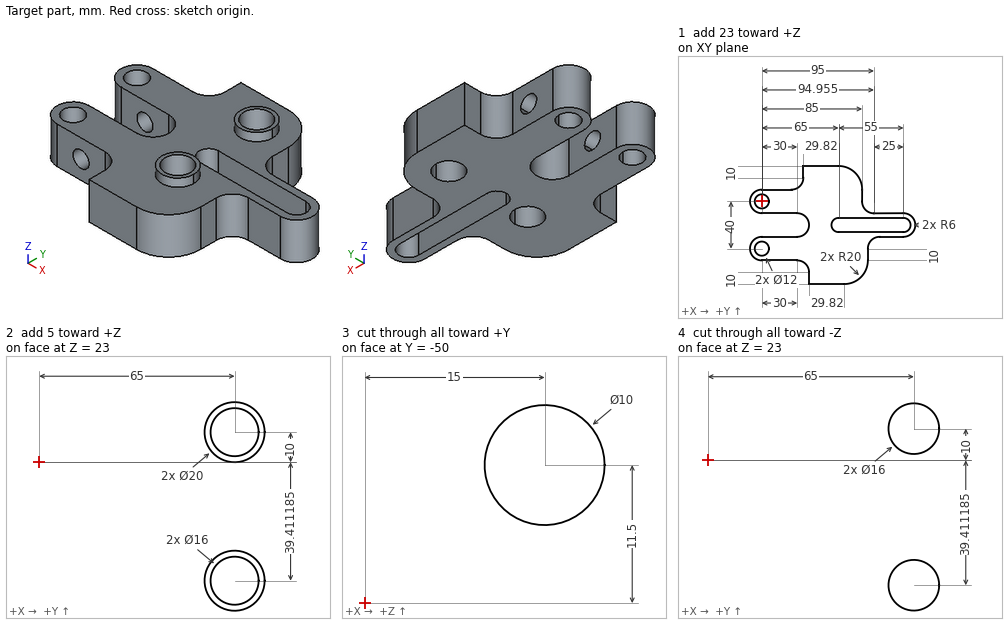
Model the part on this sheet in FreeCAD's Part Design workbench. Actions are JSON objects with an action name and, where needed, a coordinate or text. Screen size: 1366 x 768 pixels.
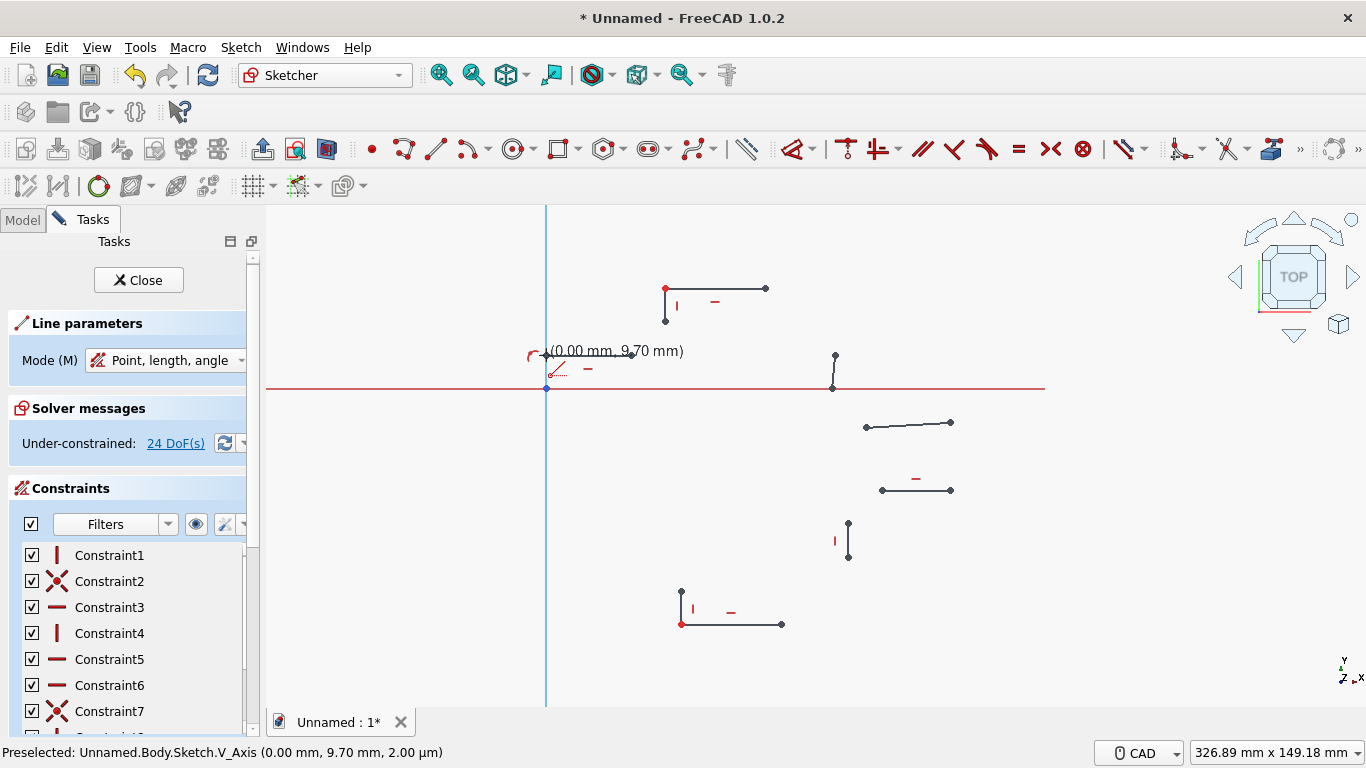
{"action": "left_click", "coordinate": [546, 422]}
{"action": "left_click", "coordinate": [647, 422]}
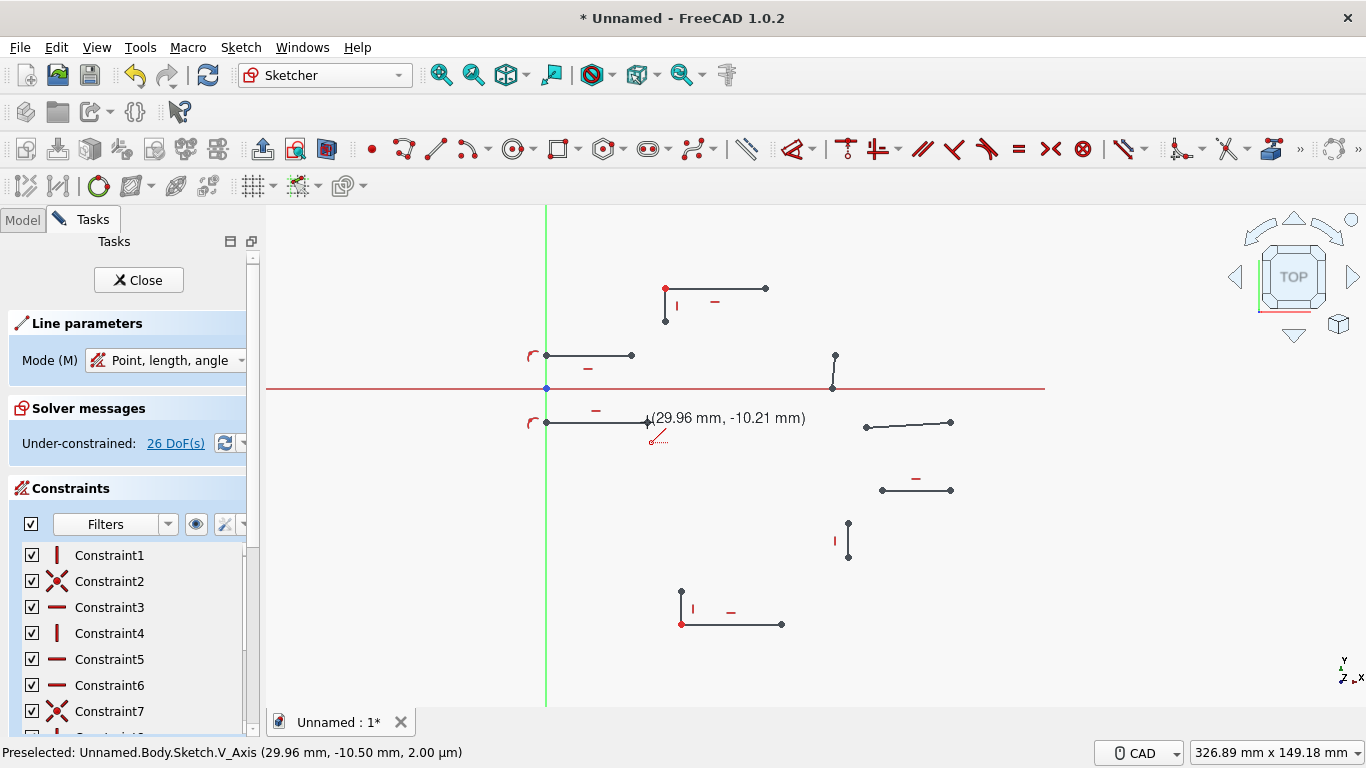
{"action": "left_click", "coordinate": [647, 490]}
{"action": "left_click", "coordinate": [546, 490]}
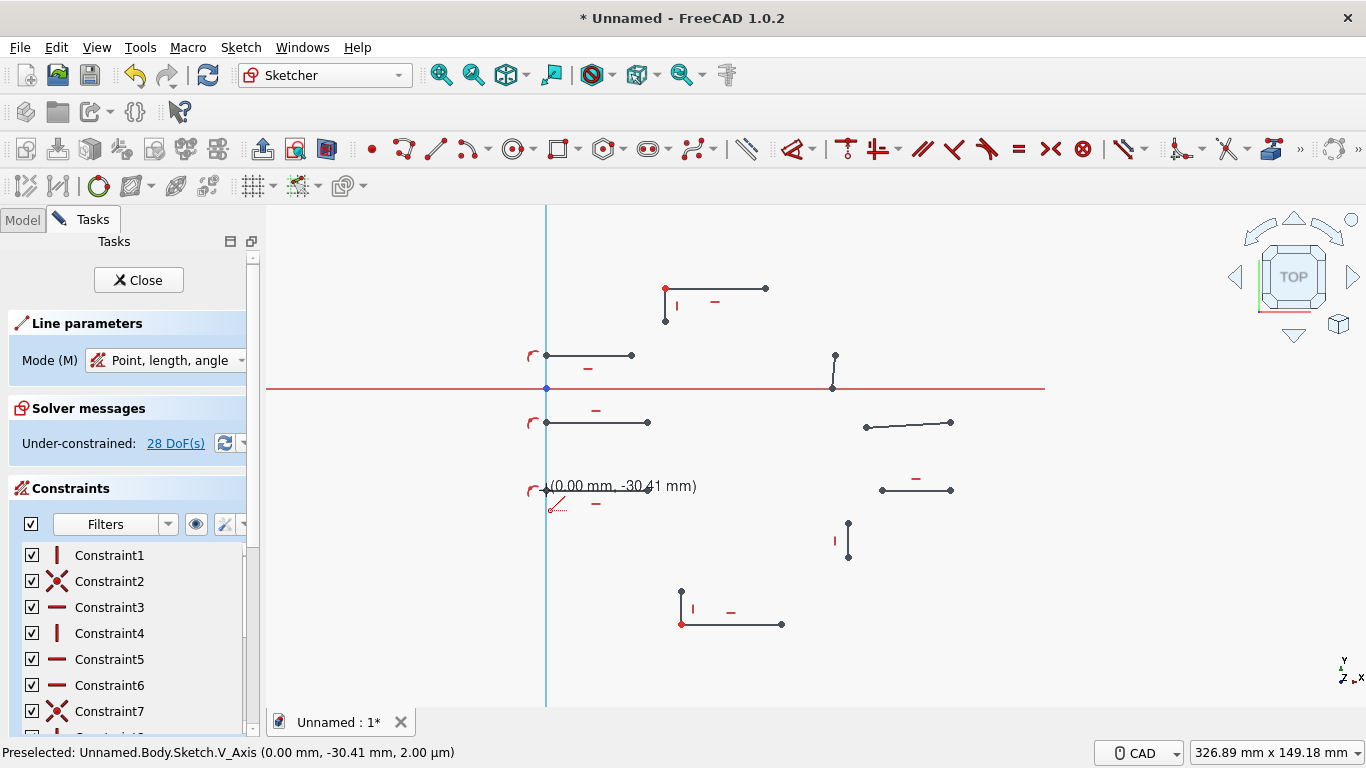
{"action": "left_click", "coordinate": [546, 557]}
{"action": "left_click", "coordinate": [647, 557]}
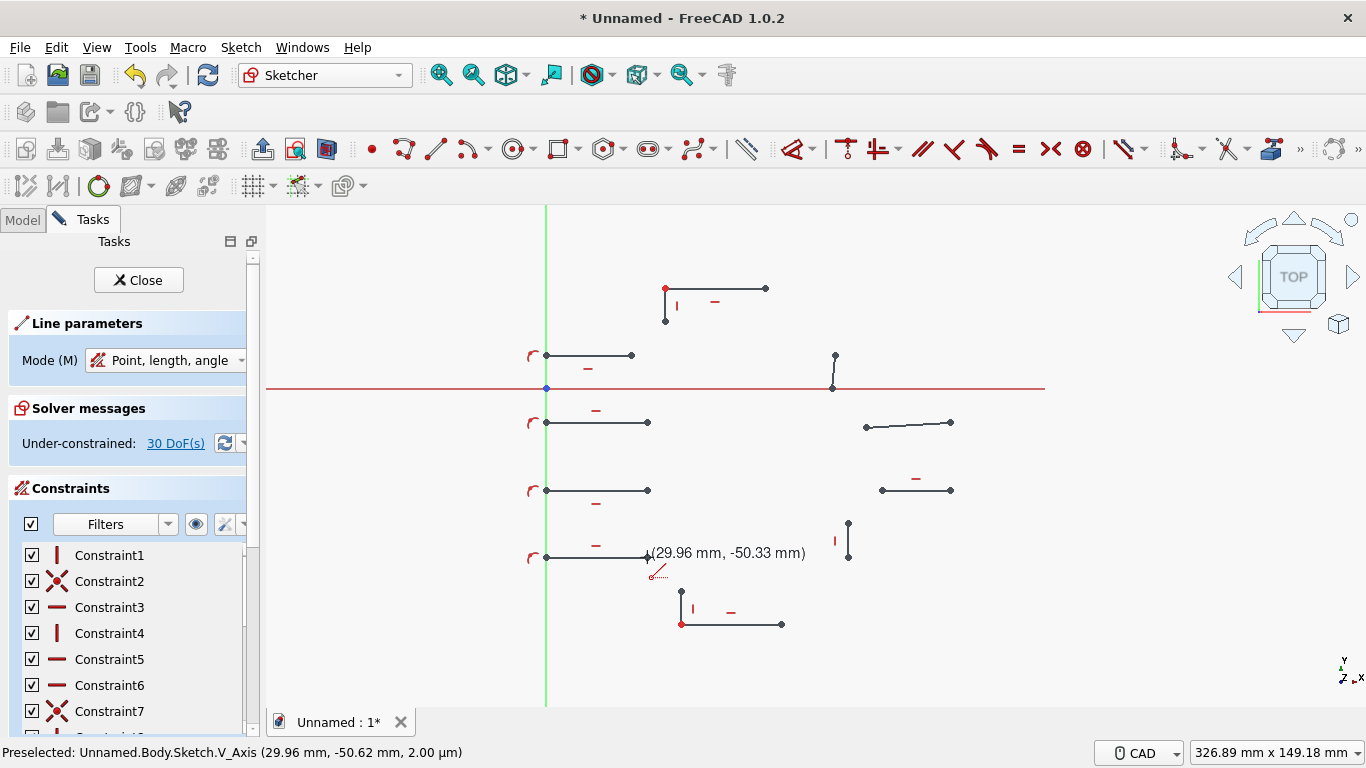
{"action": "key", "text": "g 3 a"}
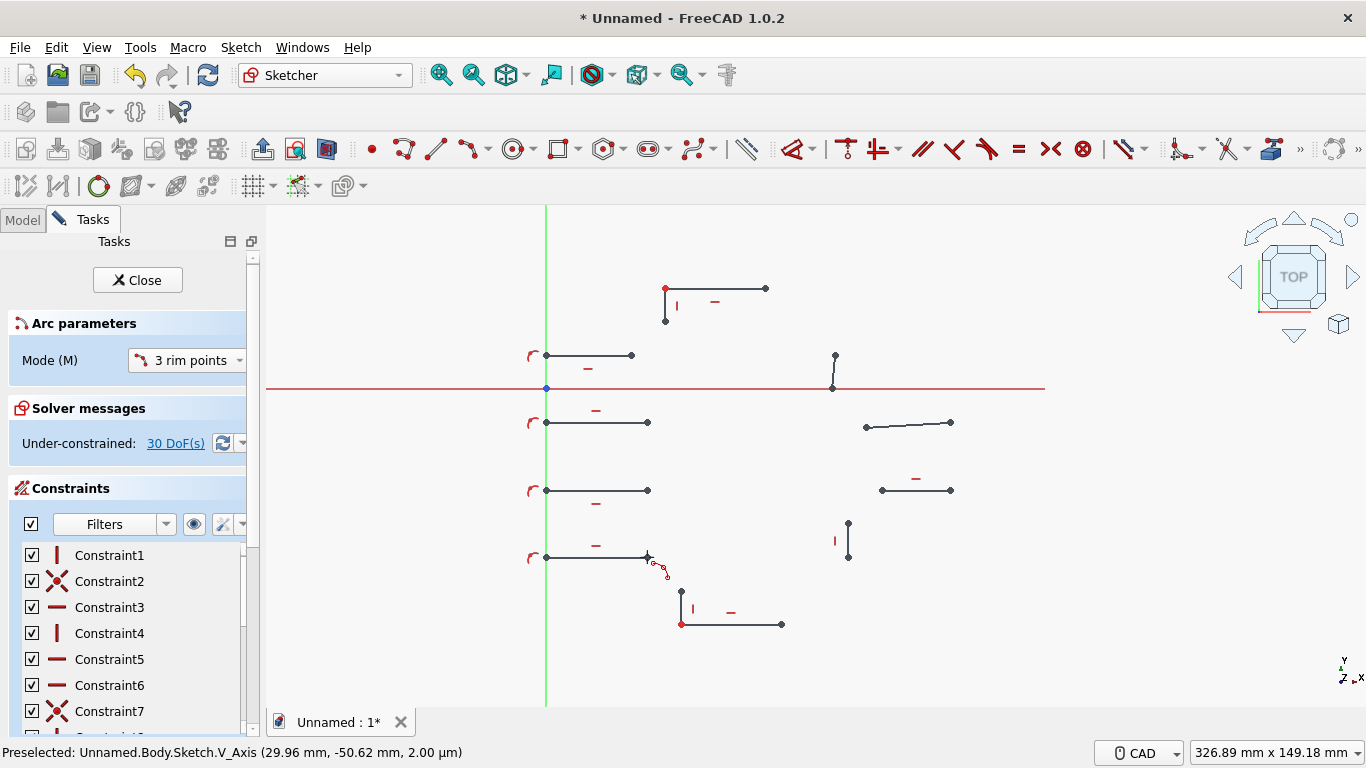
{"action": "left_click", "coordinate": [781, 625]}
{"action": "left_click", "coordinate": [848, 558]}
{"action": "left_click", "coordinate": [829, 604]}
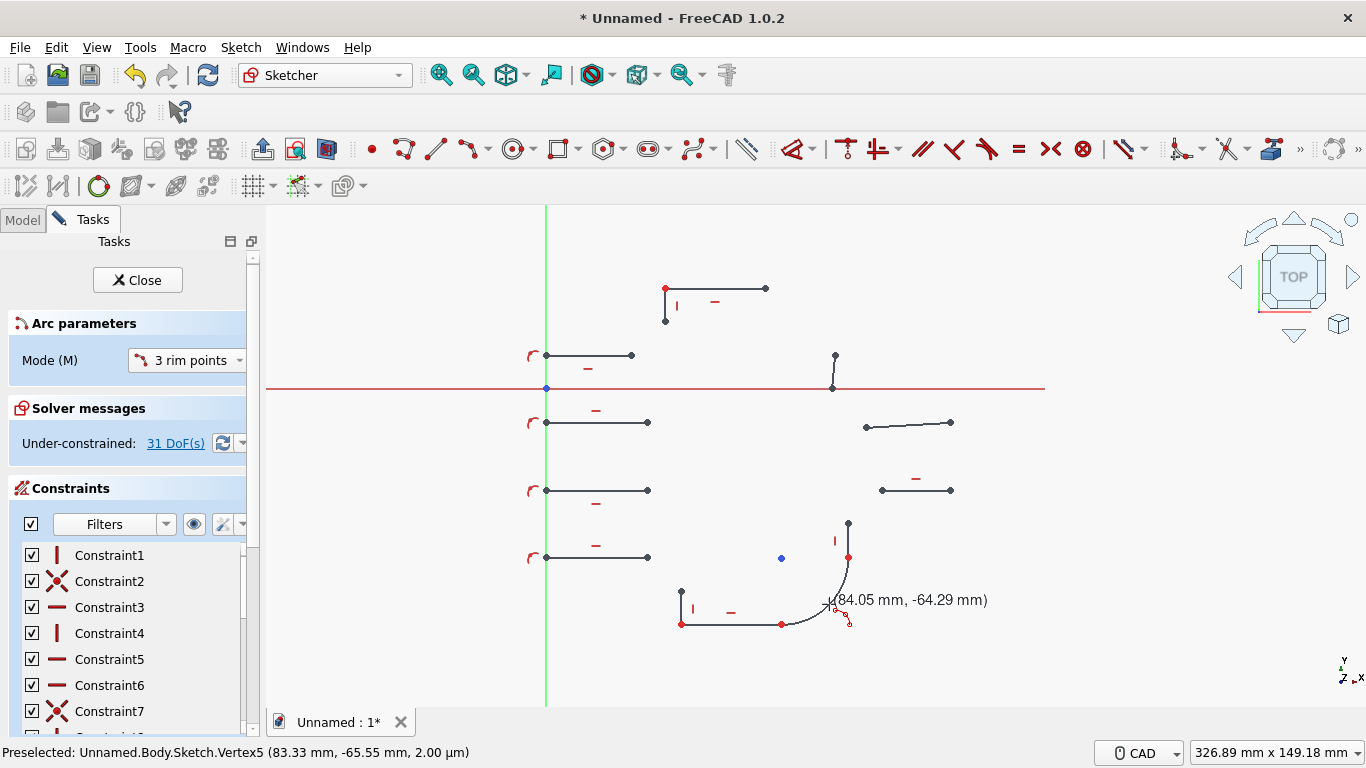
{"action": "left_click", "coordinate": [848, 524]}
{"action": "left_click", "coordinate": [882, 491]}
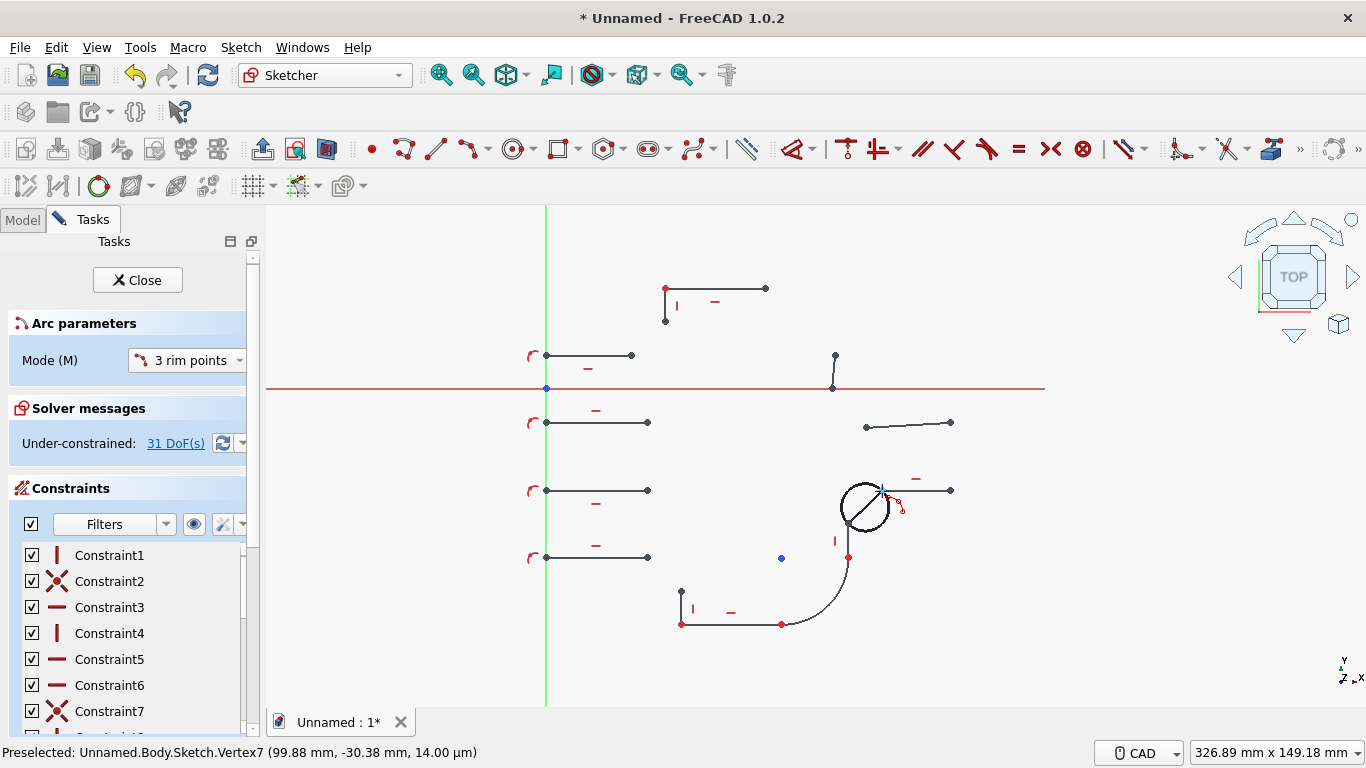
{"action": "scroll", "coordinate": [858, 499], "scroll_direction": "up", "scroll_amount": 3}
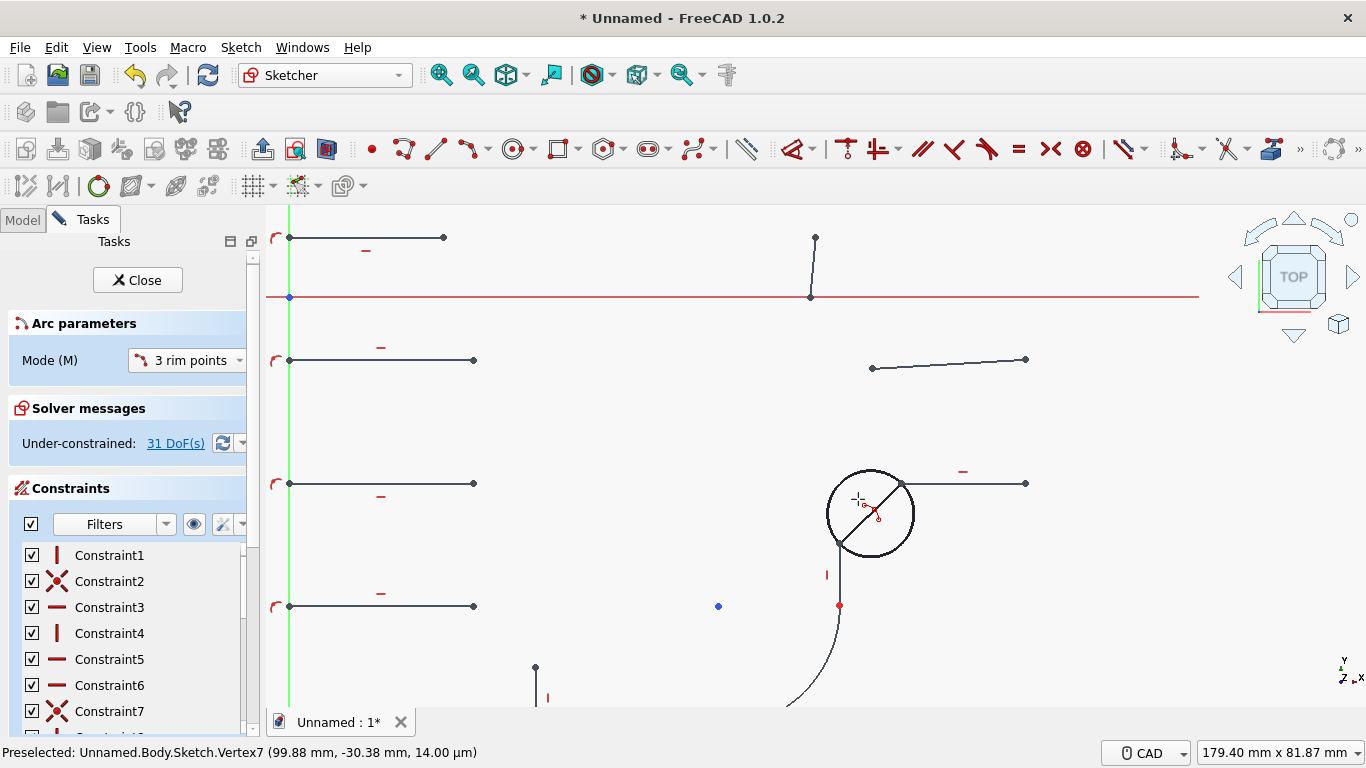
{"action": "left_click", "coordinate": [858, 499]}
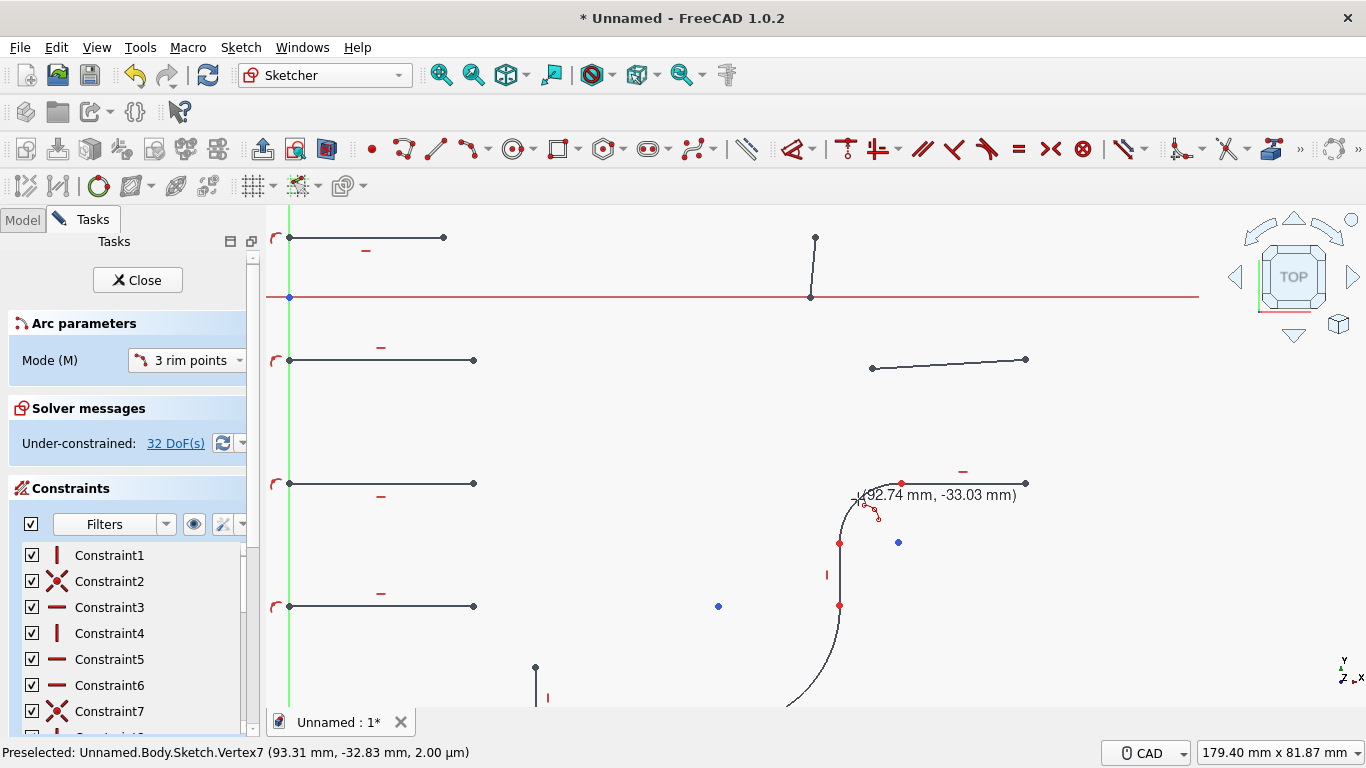
{"action": "left_click", "coordinate": [1026, 484]}
{"action": "left_click", "coordinate": [1026, 360]}
{"action": "left_click", "coordinate": [1086, 420]}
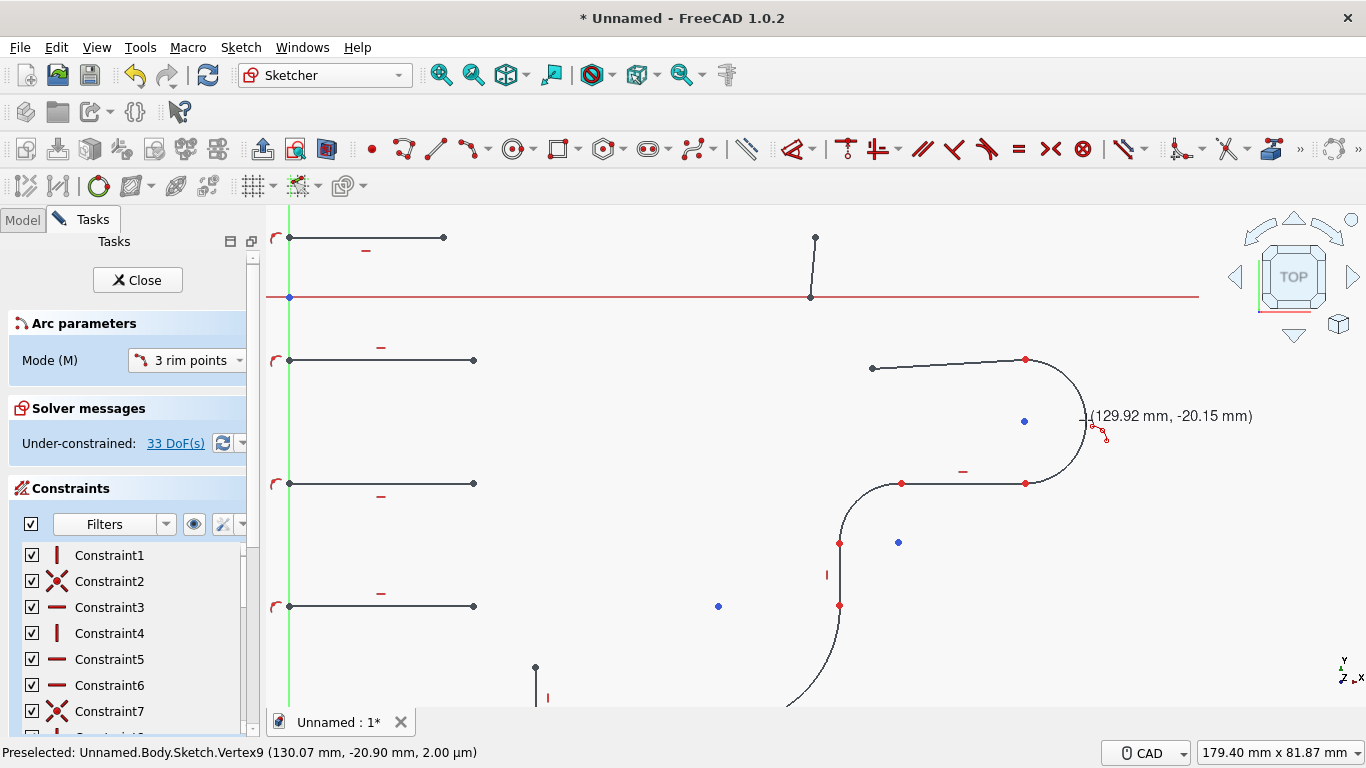
{"action": "left_click", "coordinate": [873, 369]}